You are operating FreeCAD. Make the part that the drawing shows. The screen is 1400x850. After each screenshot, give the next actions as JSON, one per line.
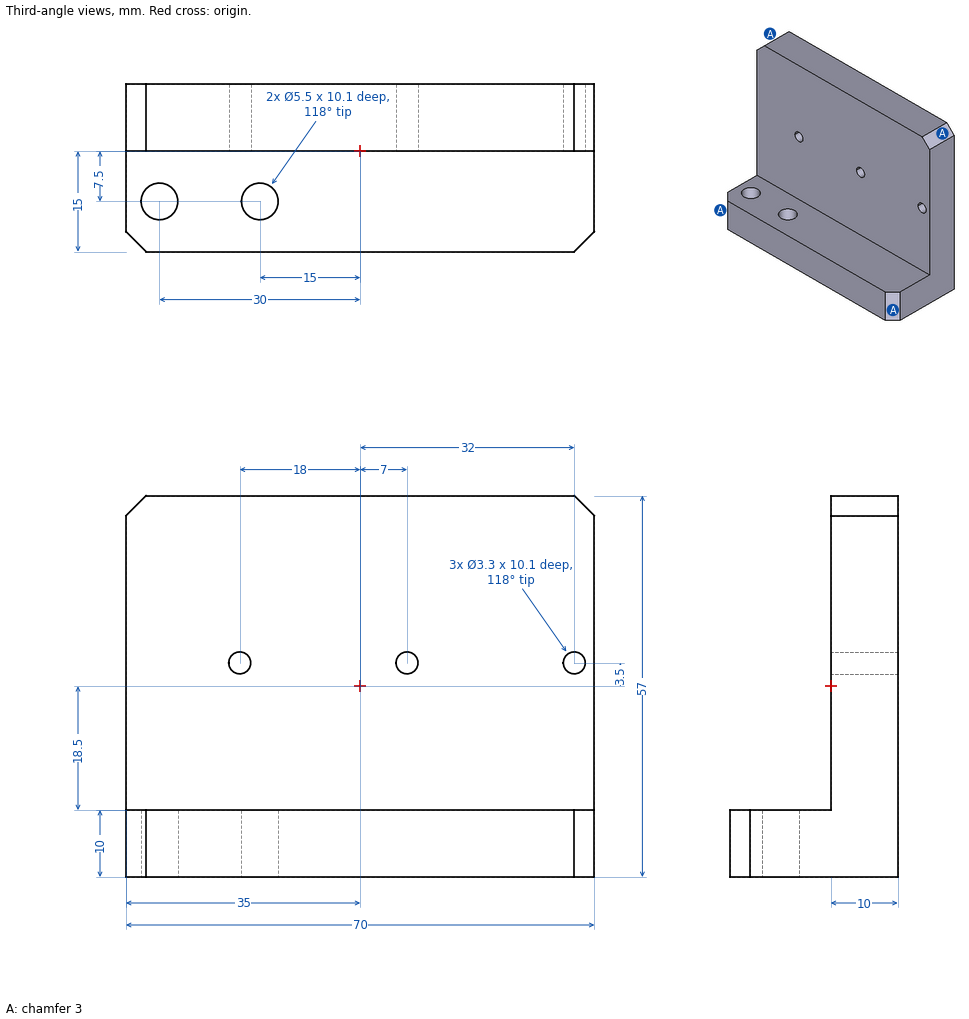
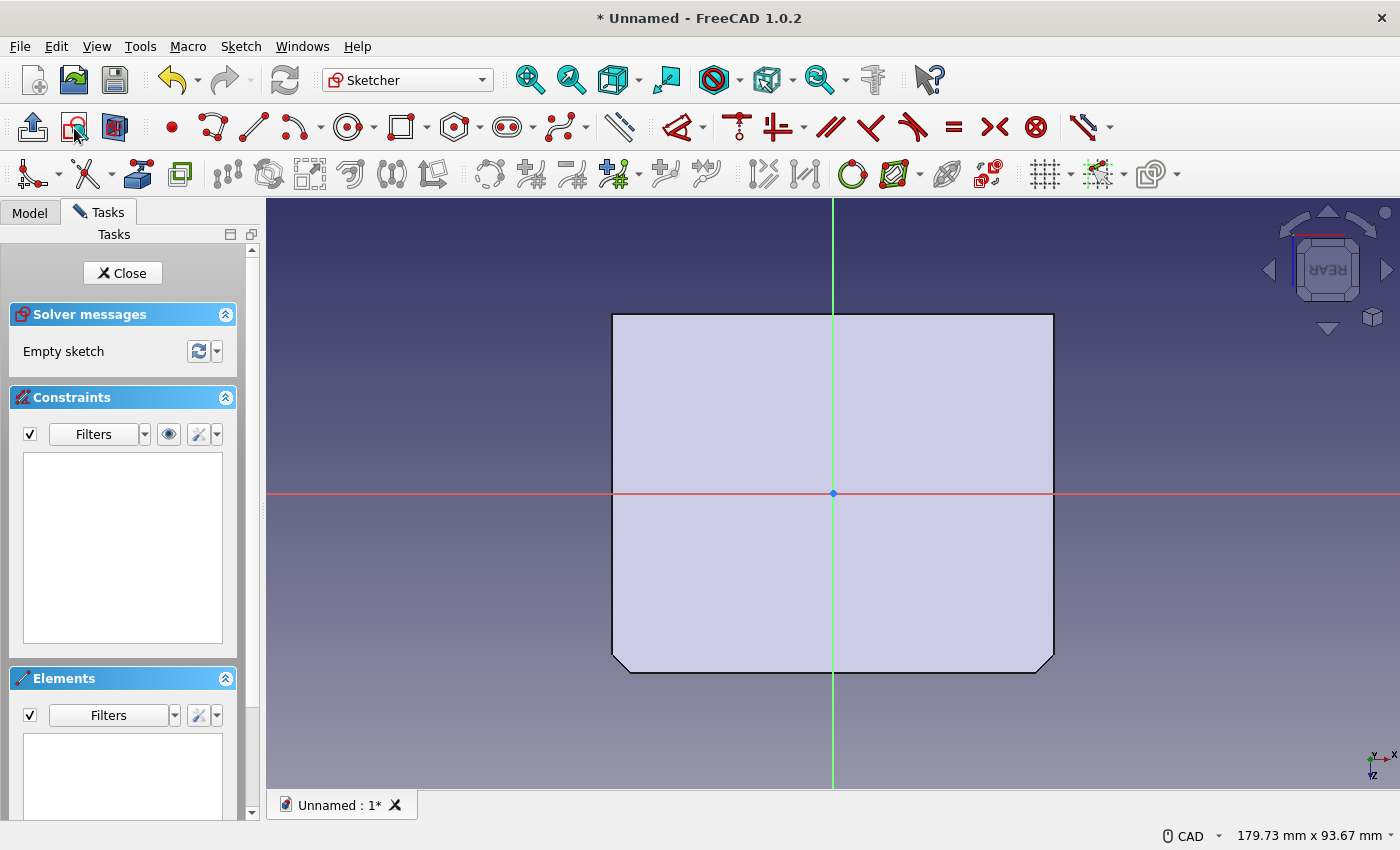
{"action": "scroll", "coordinate": [1014, 530], "scroll_direction": "up", "scroll_amount": 3}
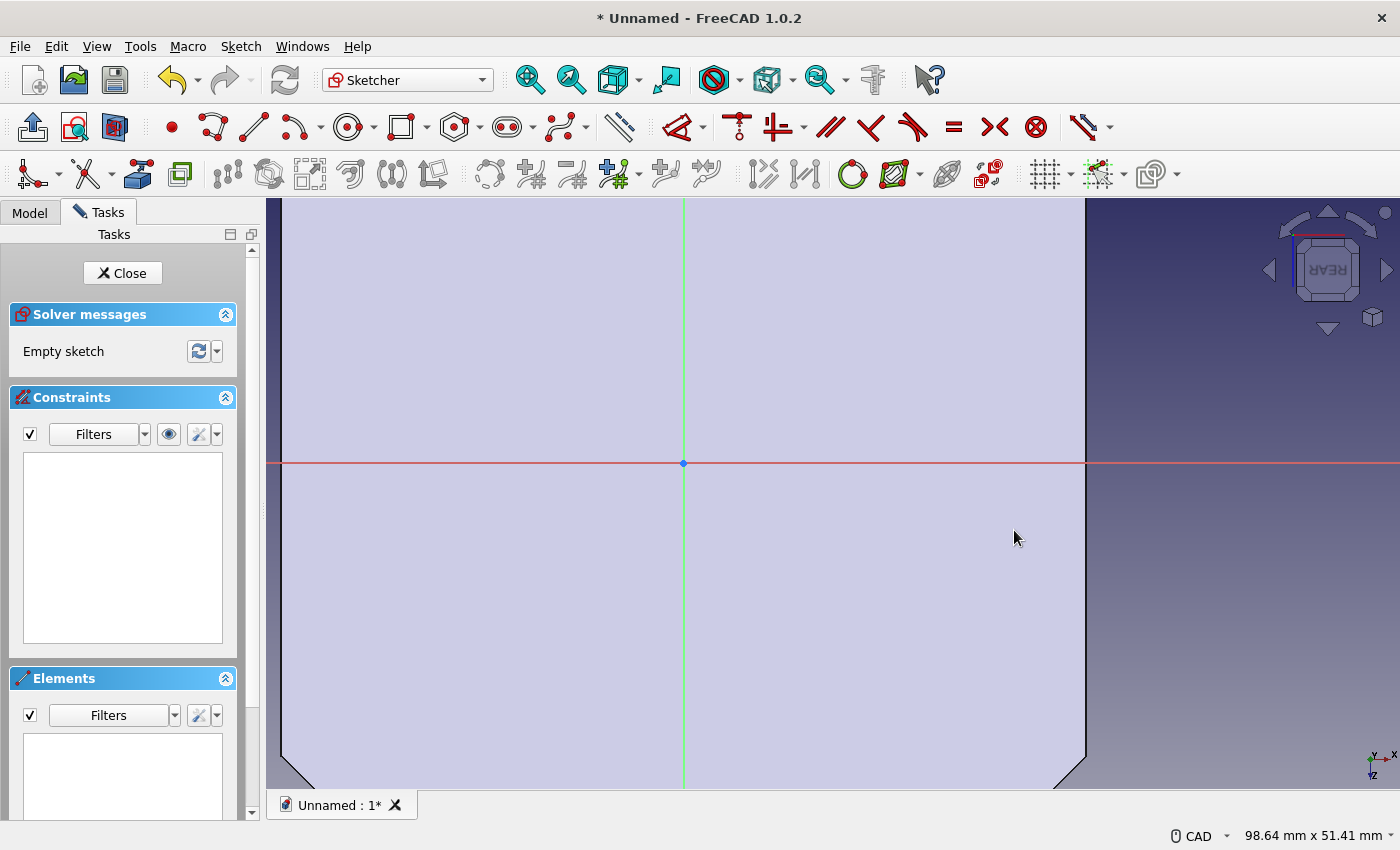
{"action": "left_click", "coordinate": [348, 128]}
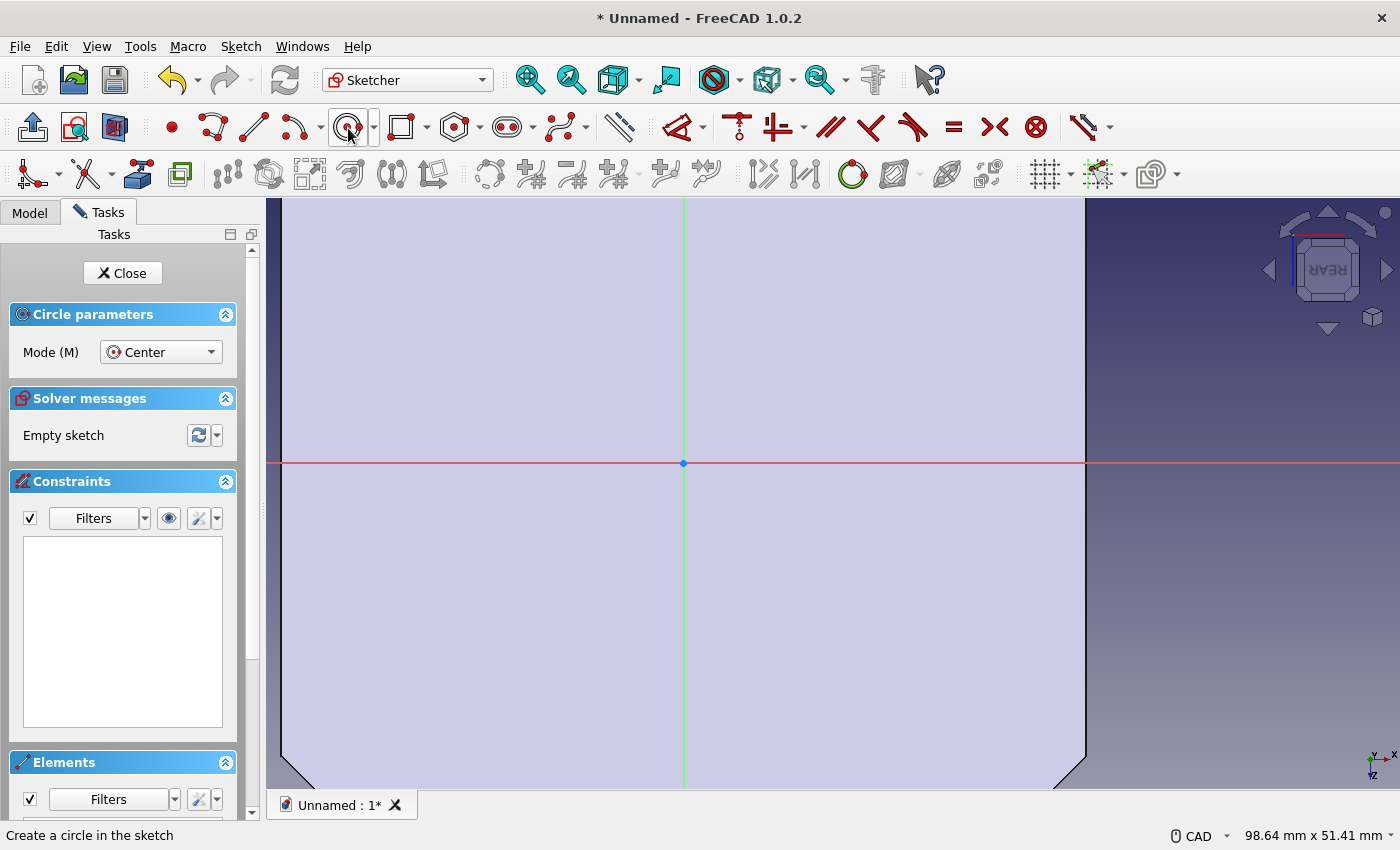
{"action": "left_click", "coordinate": [1052, 503]}
{"action": "left_click", "coordinate": [1065, 490]}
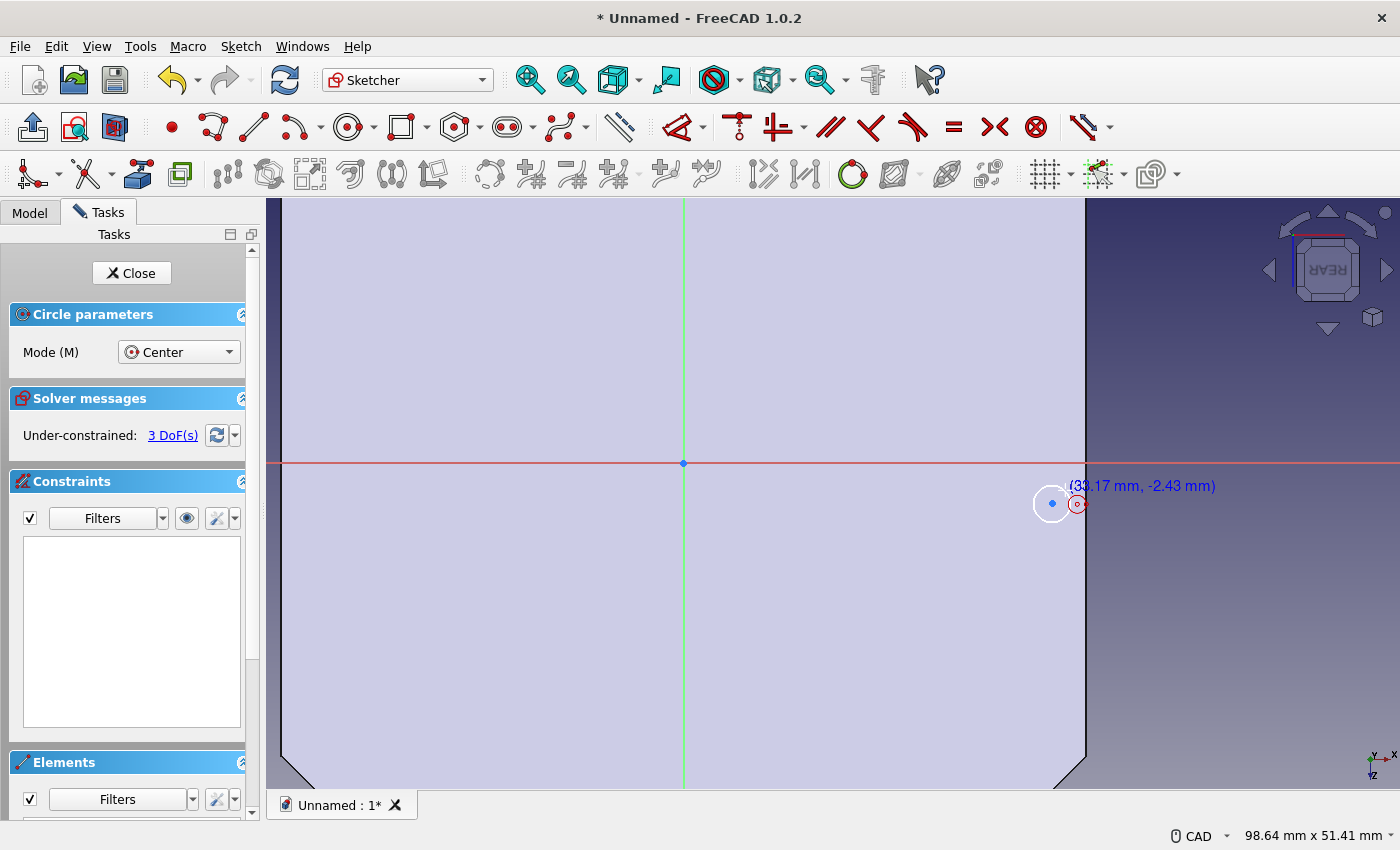
{"action": "left_click", "coordinate": [477, 503]}
{"action": "left_click", "coordinate": [490, 490]}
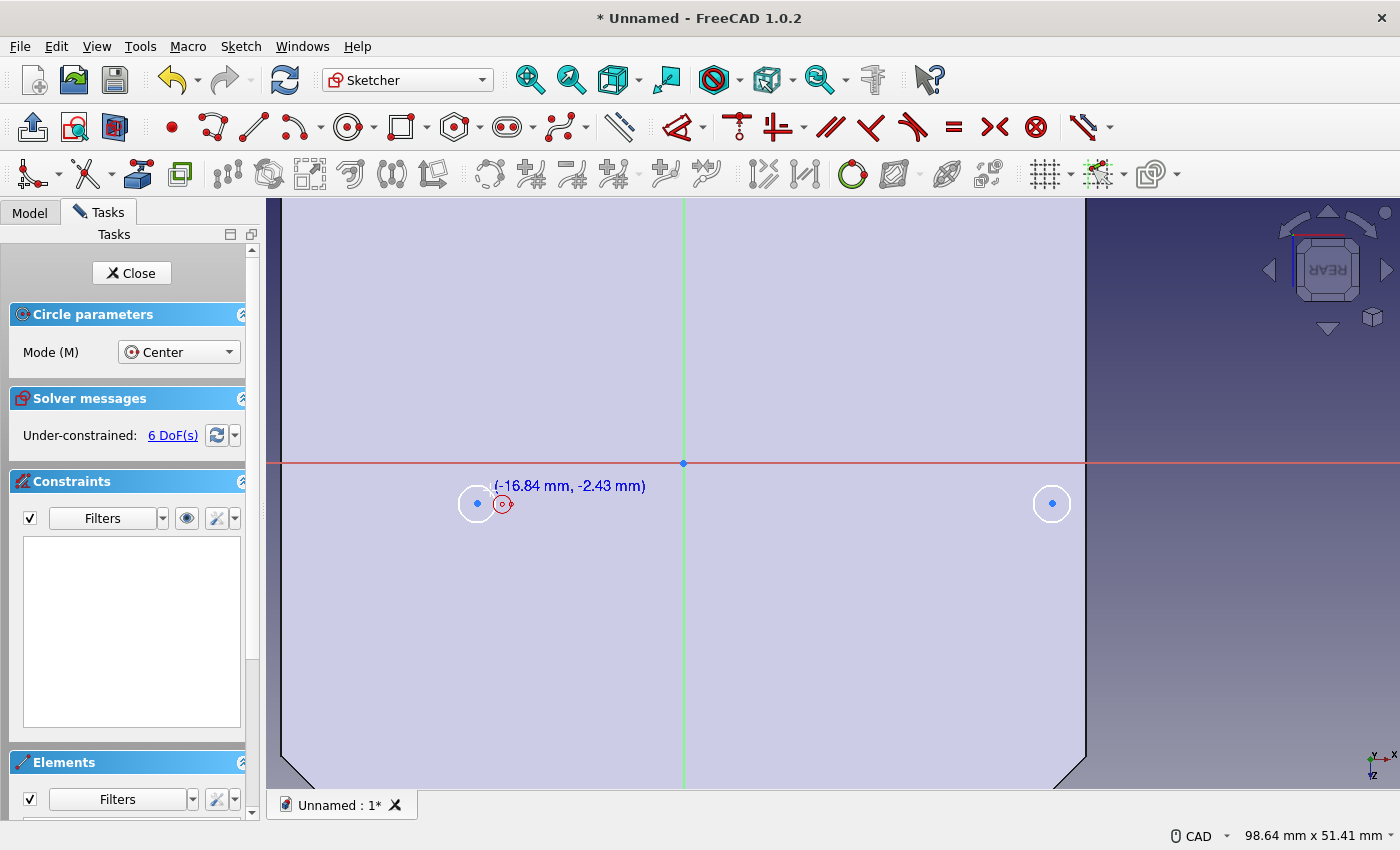
{"action": "left_click", "coordinate": [764, 503]}
{"action": "left_click", "coordinate": [778, 490]}
{"action": "key", "text": "Escape"}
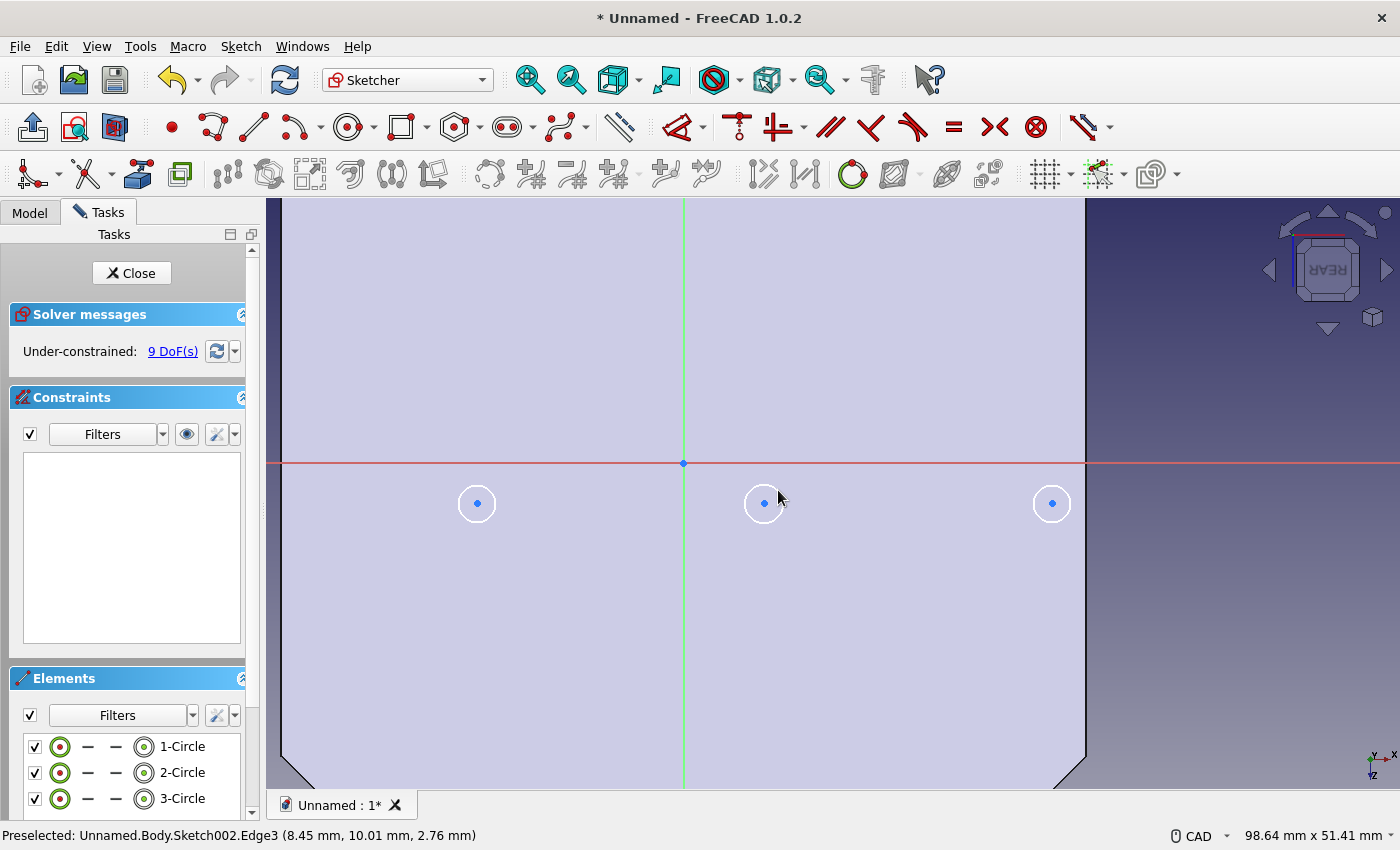
{"action": "left_click", "coordinate": [1065, 491]}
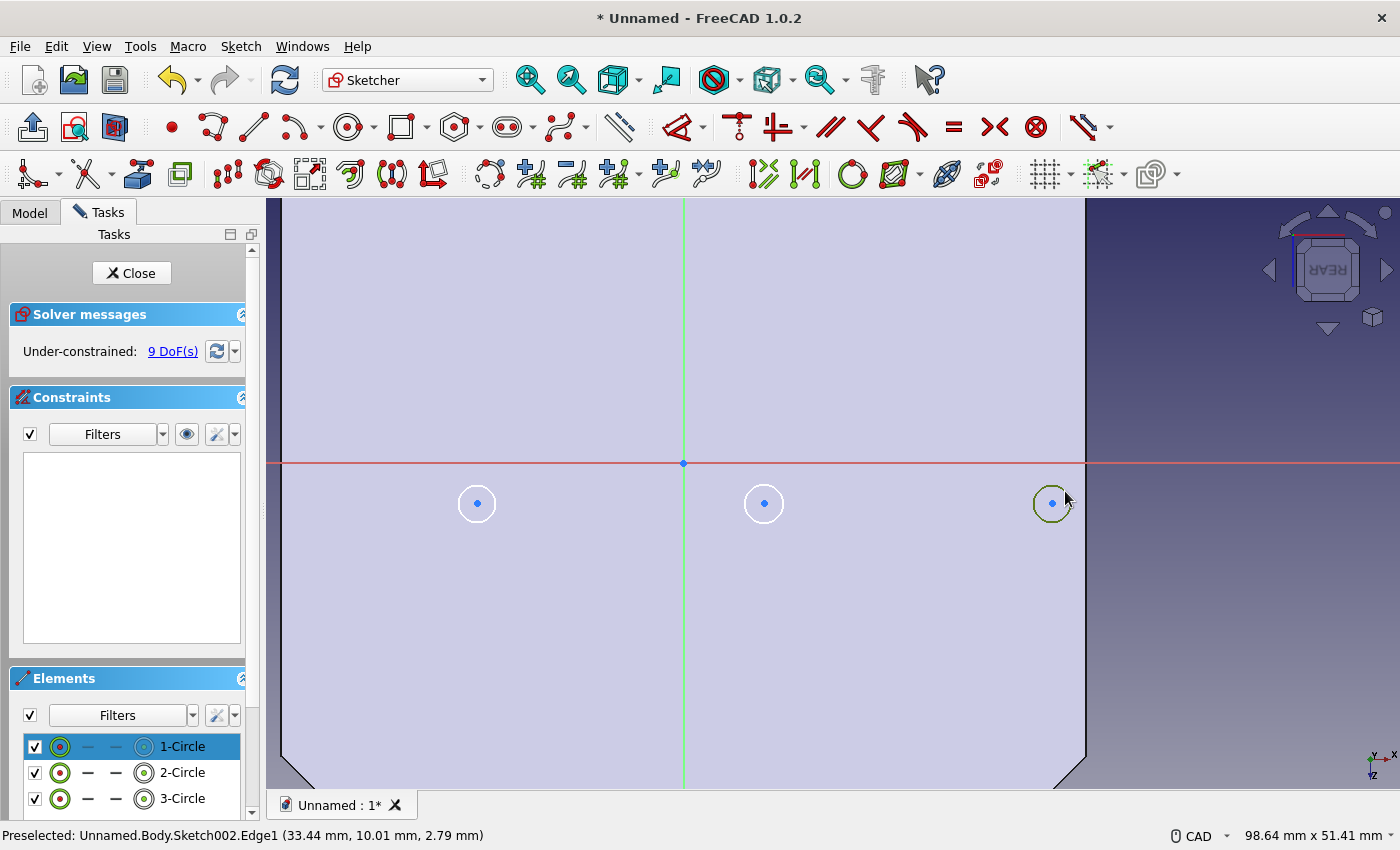
{"action": "left_click", "coordinate": [490, 491]}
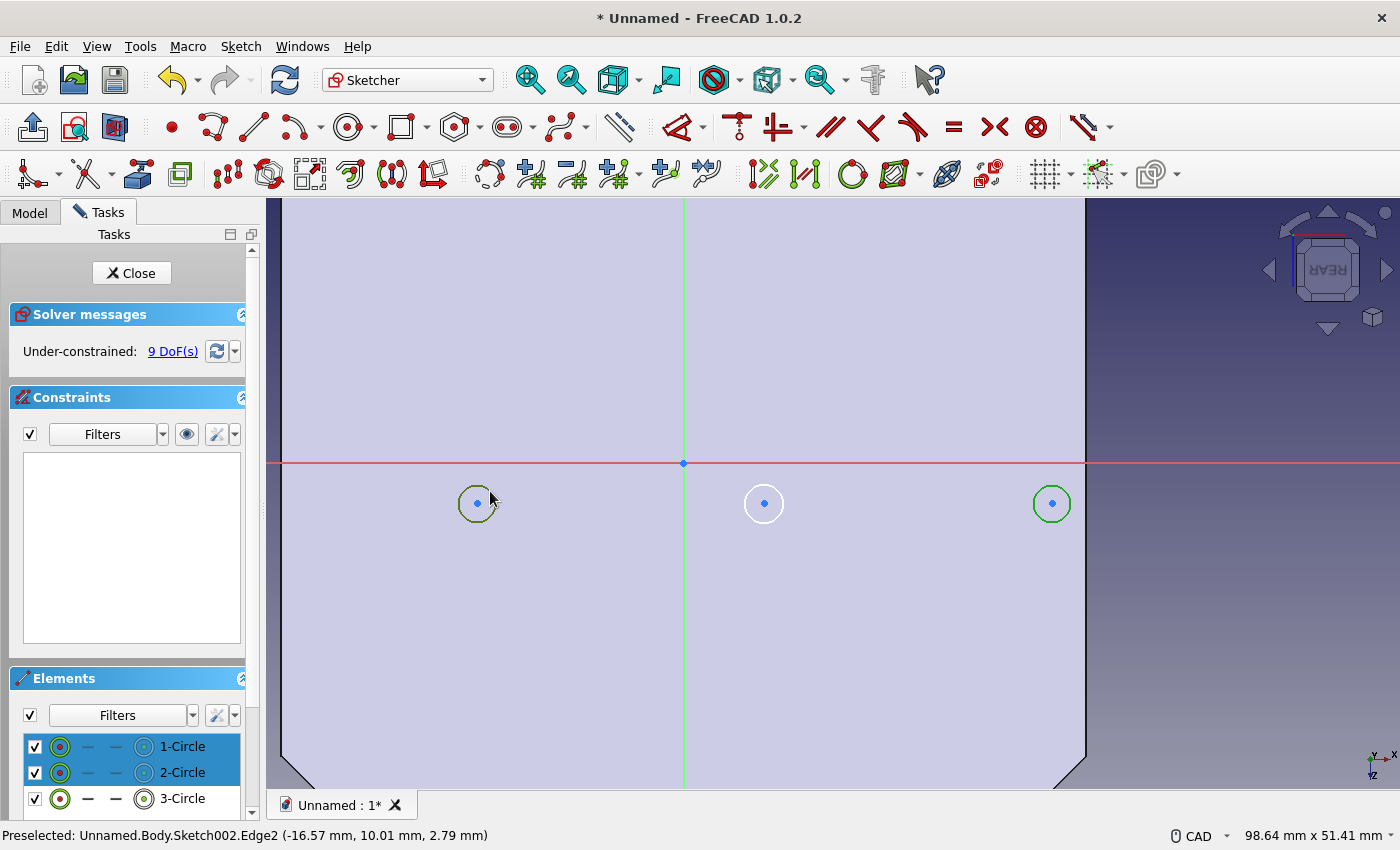
{"action": "left_click", "coordinate": [777, 490]}